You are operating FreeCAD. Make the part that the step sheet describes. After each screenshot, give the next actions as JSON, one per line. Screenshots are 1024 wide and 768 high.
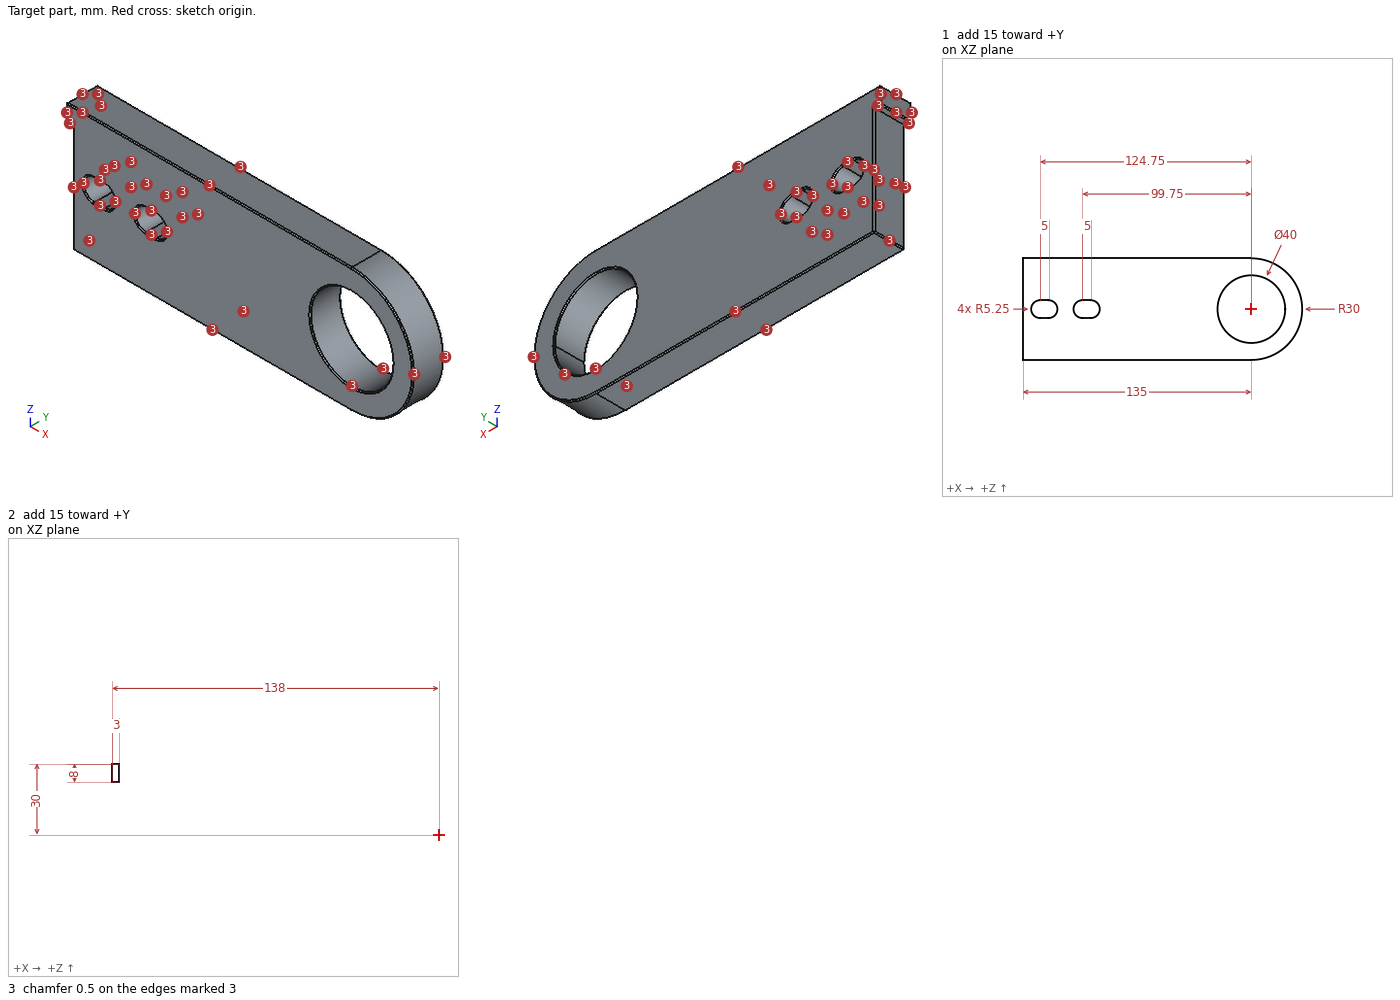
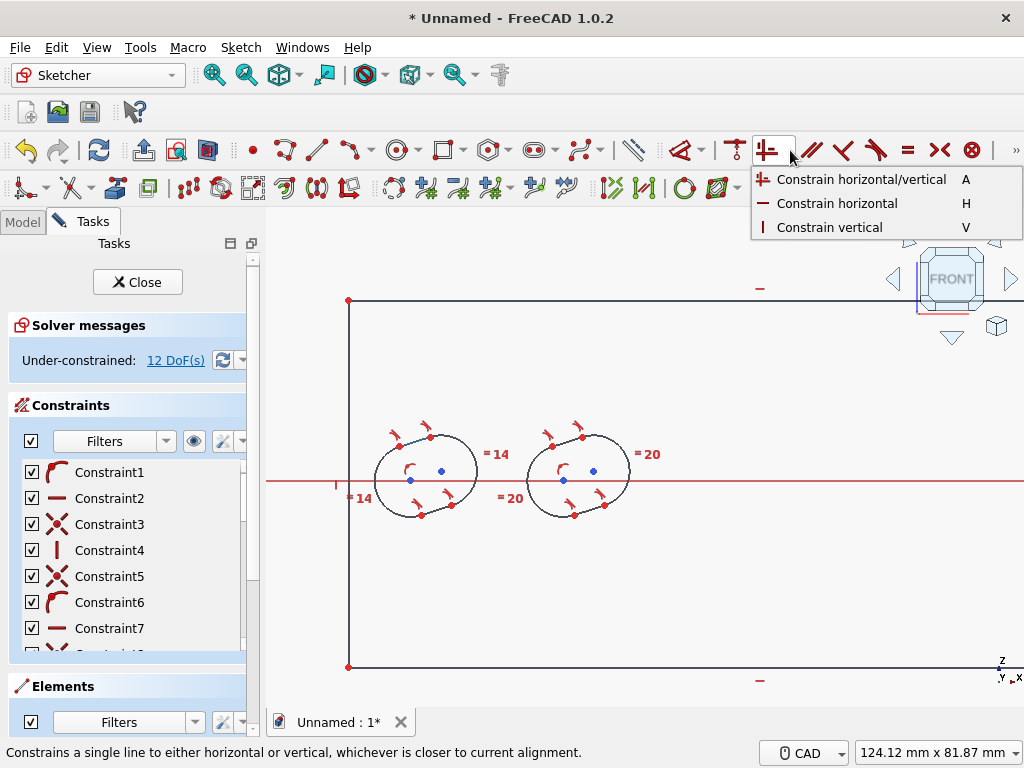
{"action": "left_click", "coordinate": [887, 203]}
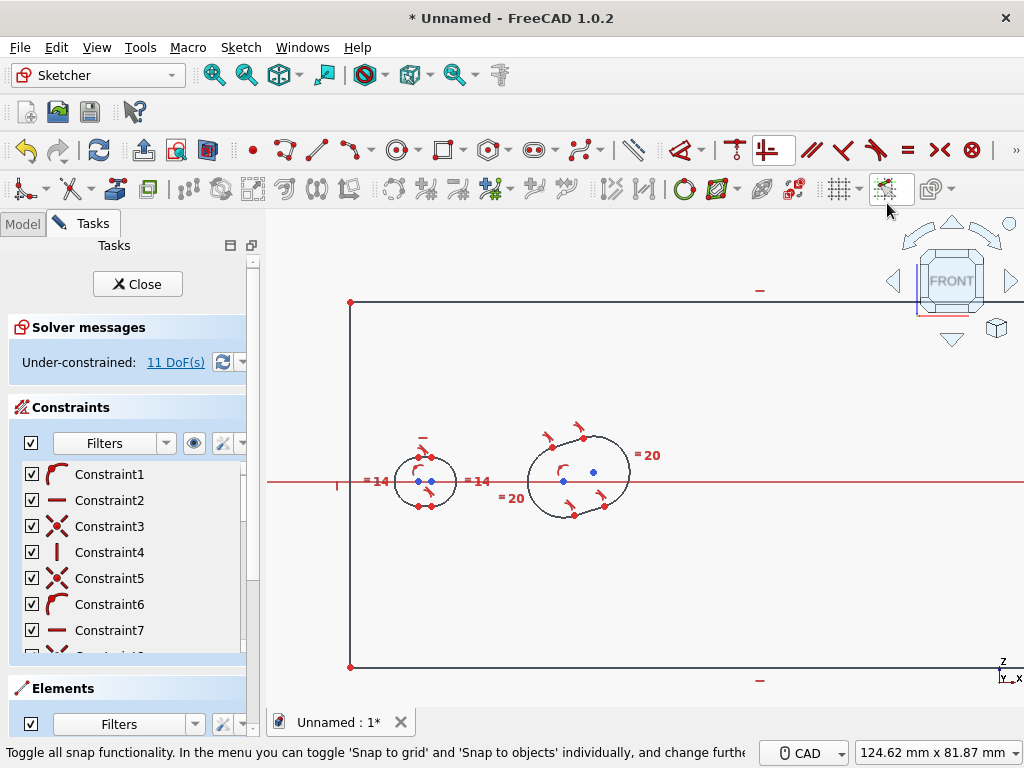
{"action": "scroll", "coordinate": [562, 445], "scroll_direction": "up", "scroll_amount": 2}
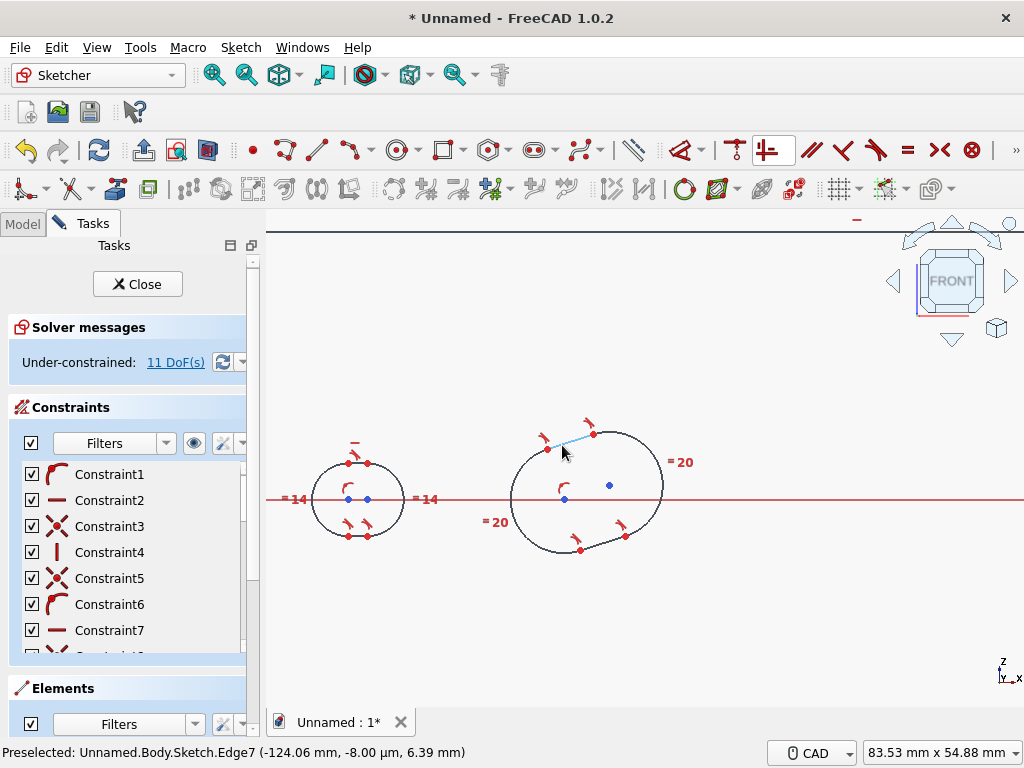
{"action": "left_click", "coordinate": [561, 445]}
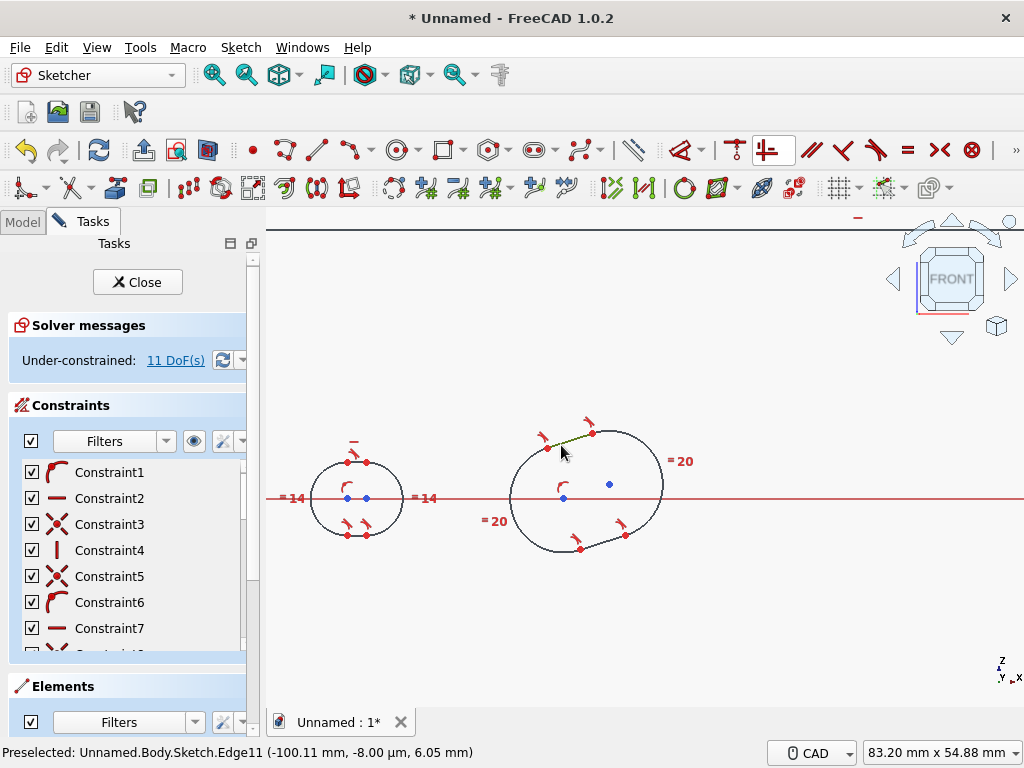
{"action": "key", "text": "h"}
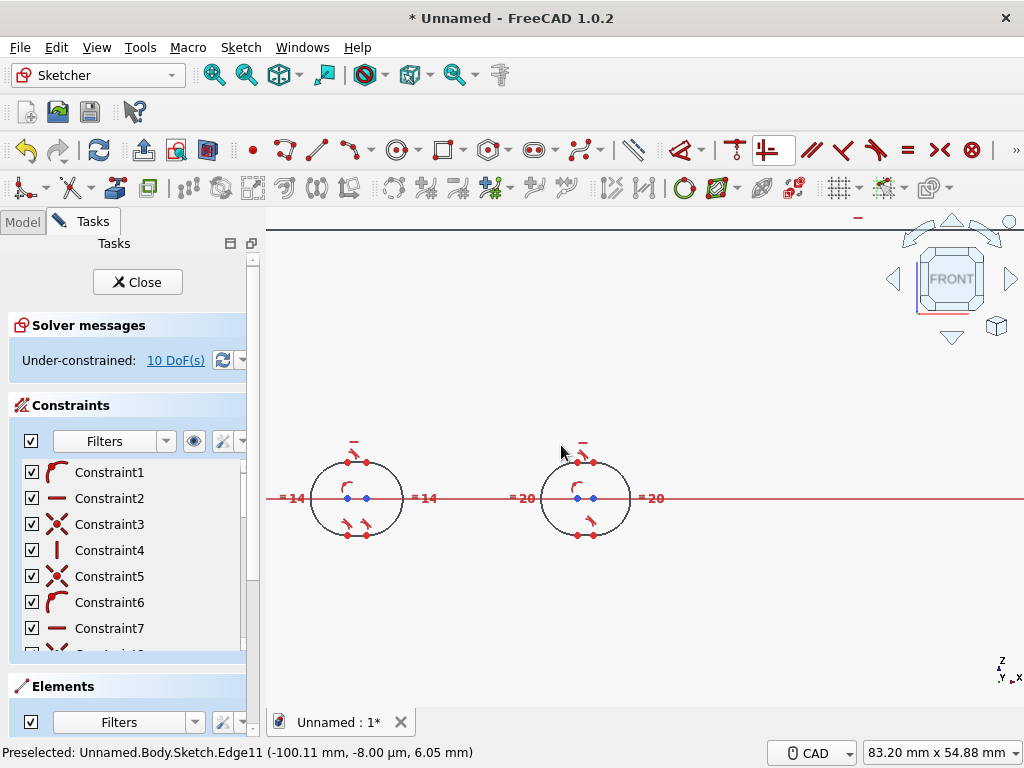
{"action": "scroll", "coordinate": [440, 443], "scroll_direction": "down", "scroll_amount": 7}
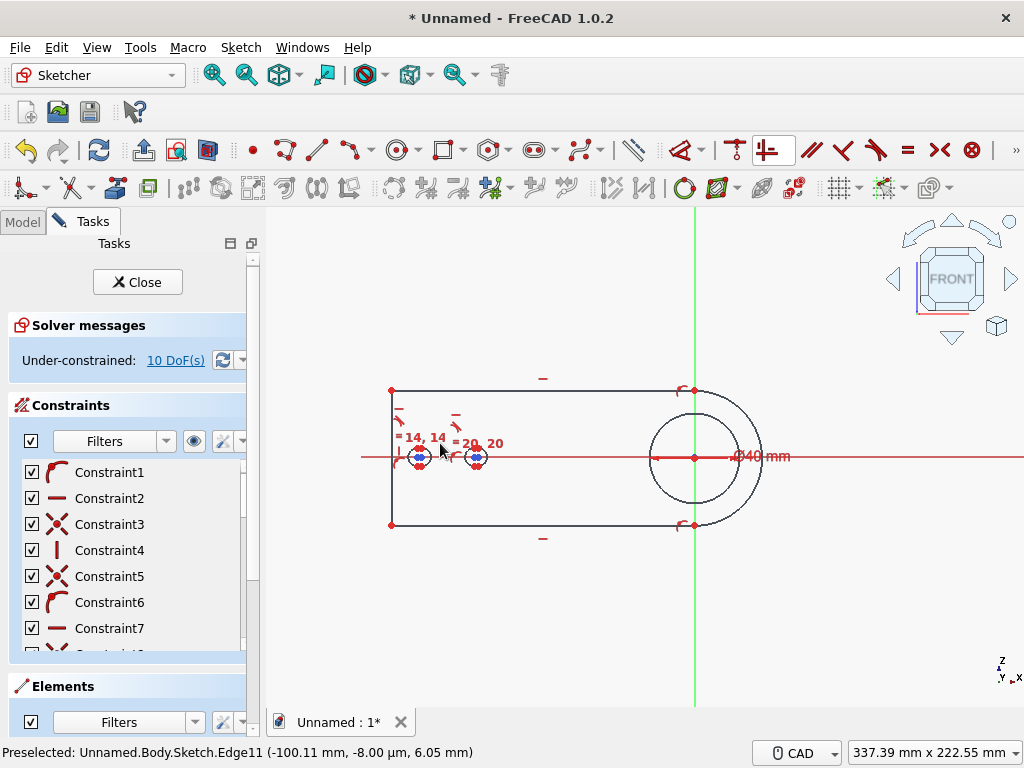
{"action": "scroll", "coordinate": [695, 458], "scroll_direction": "up", "scroll_amount": 8}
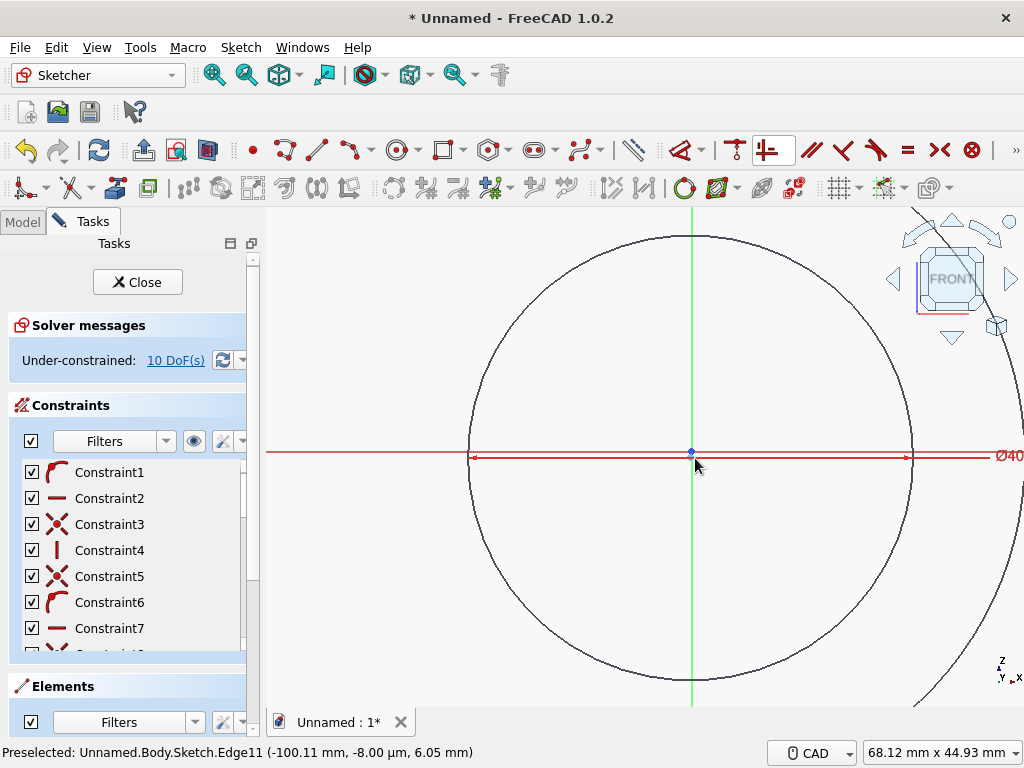
{"action": "left_click_drag", "start_coordinate": [681, 442], "coordinate": [702, 468]}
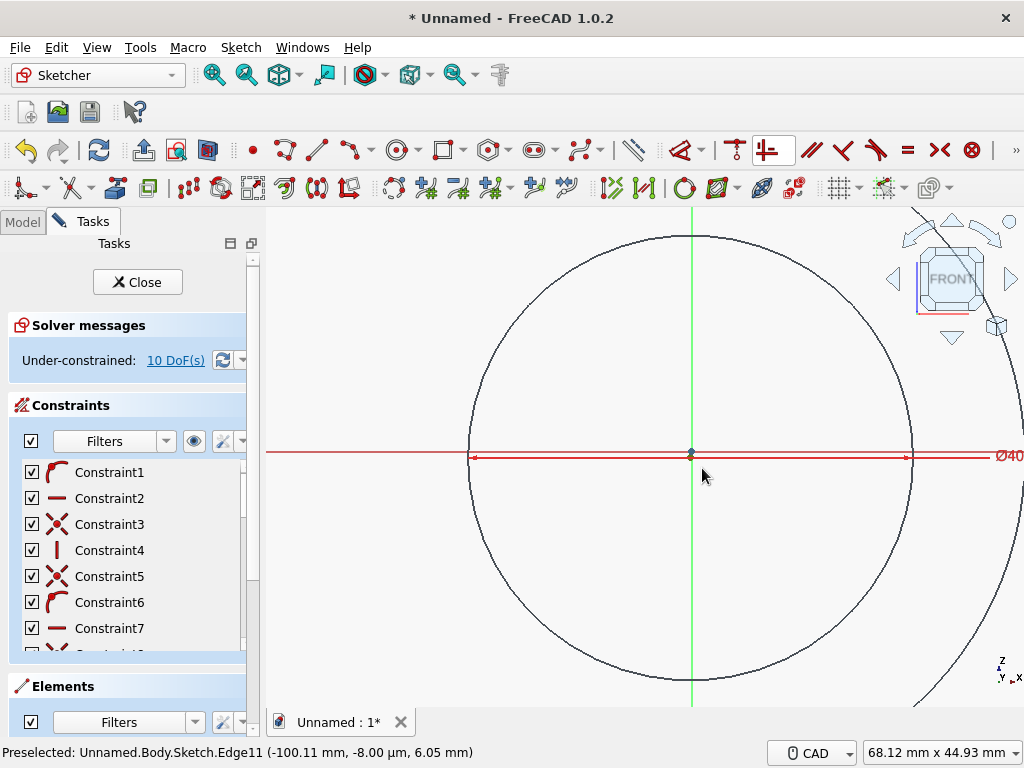
{"action": "left_click", "coordinate": [736, 150]}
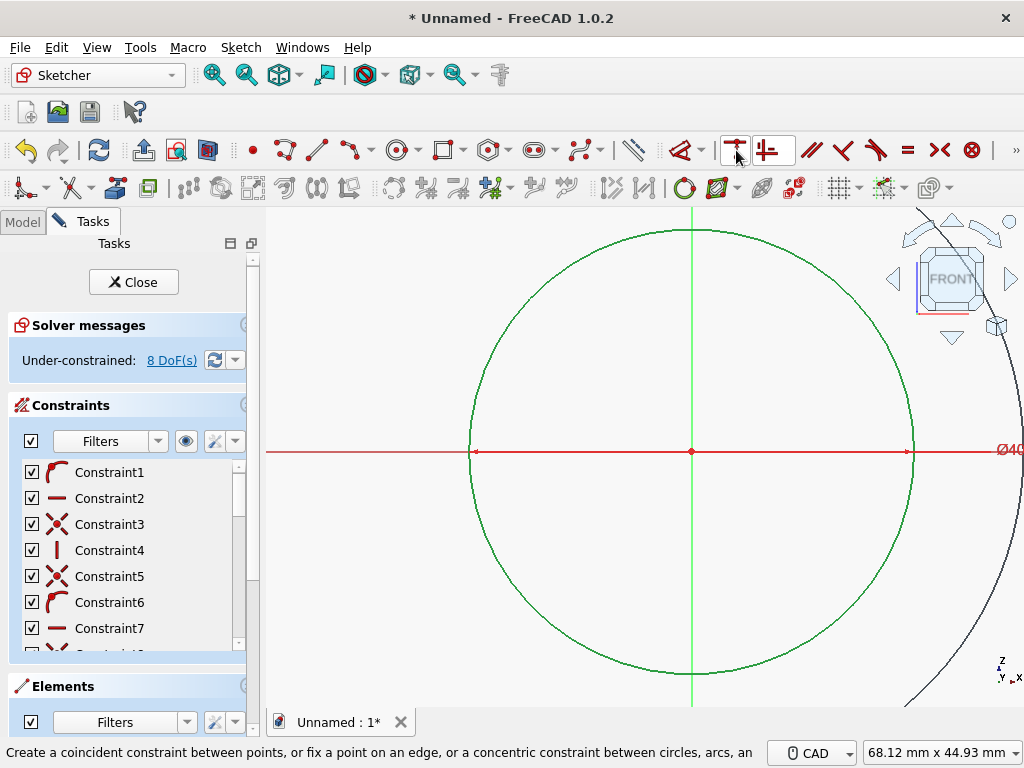
{"action": "scroll", "coordinate": [695, 458], "scroll_direction": "down", "scroll_amount": 8}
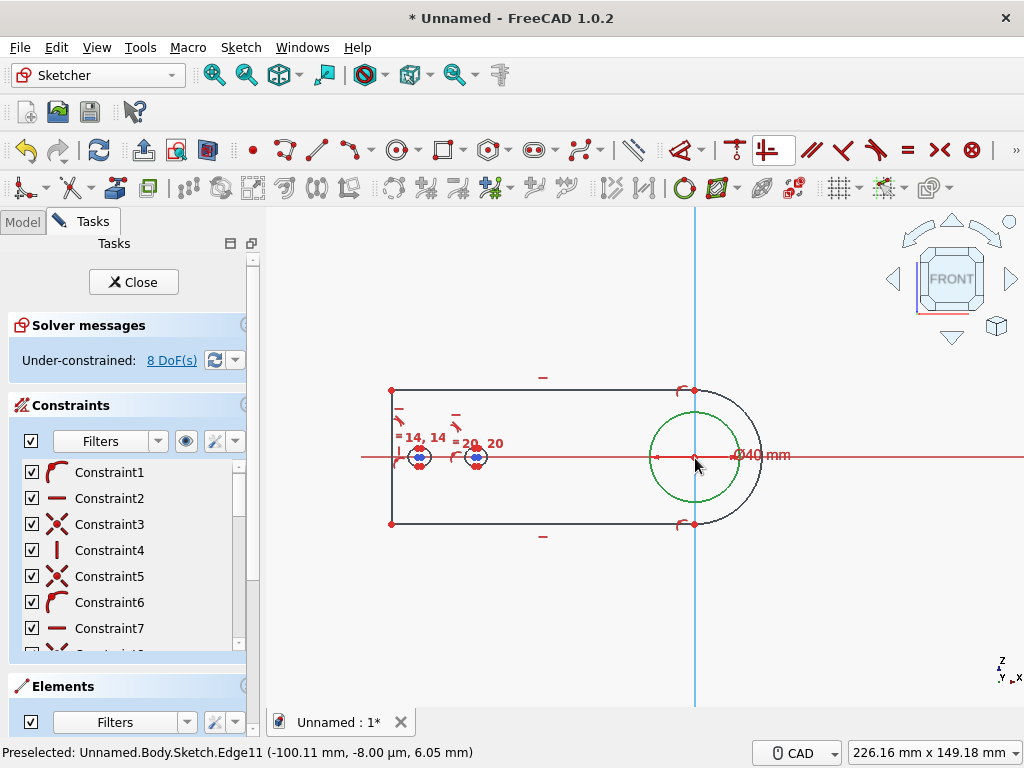
{"action": "scroll", "coordinate": [410, 452], "scroll_direction": "up", "scroll_amount": 5}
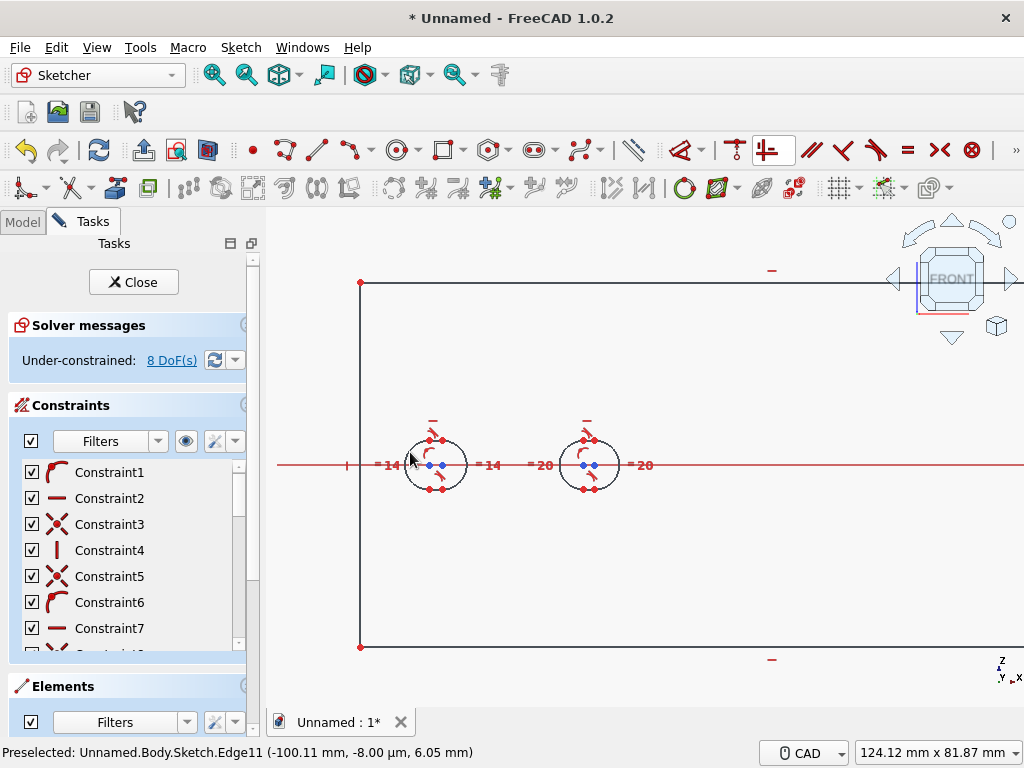
{"action": "left_click", "coordinate": [410, 451]}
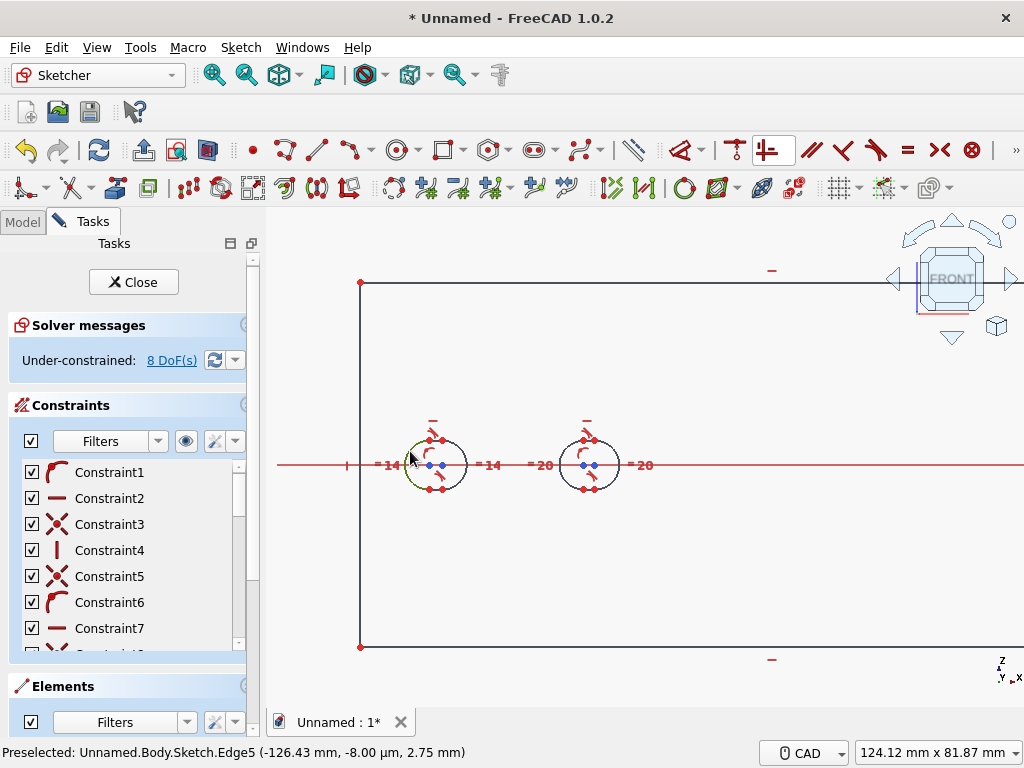
{"action": "left_click", "coordinate": [564, 451]}